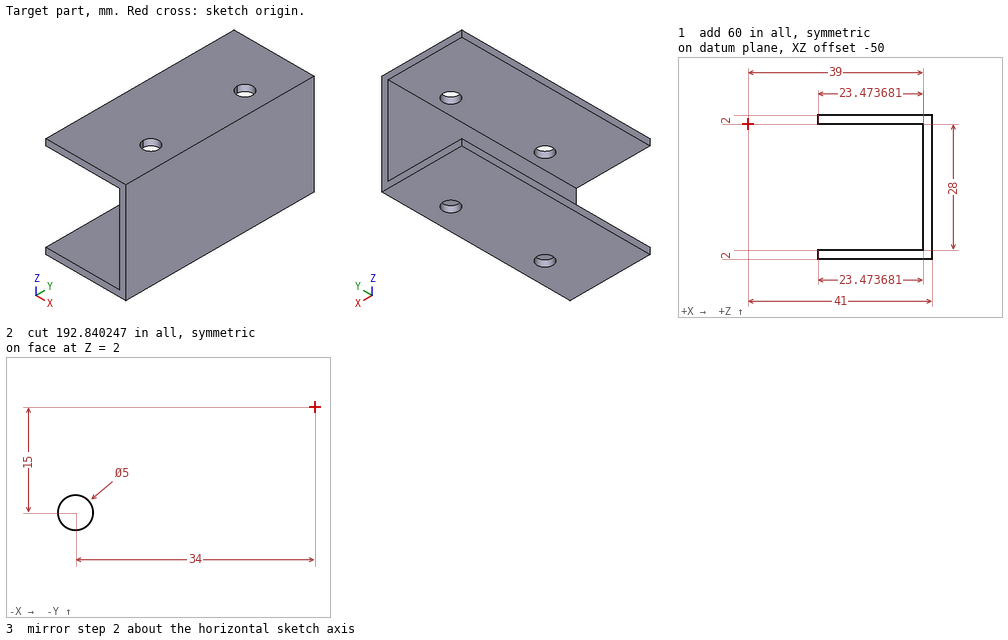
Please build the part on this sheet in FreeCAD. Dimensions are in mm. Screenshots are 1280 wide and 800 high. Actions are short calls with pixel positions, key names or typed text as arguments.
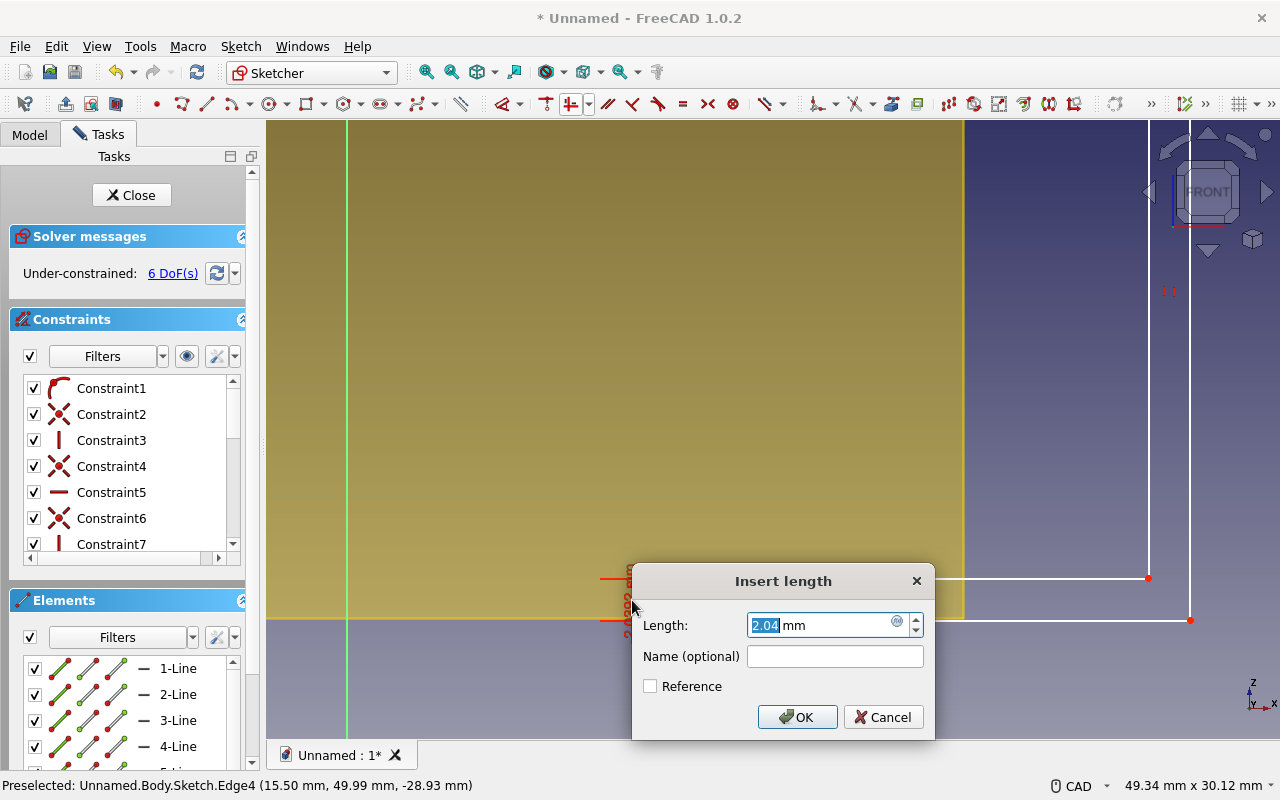
text(2)
key(Return)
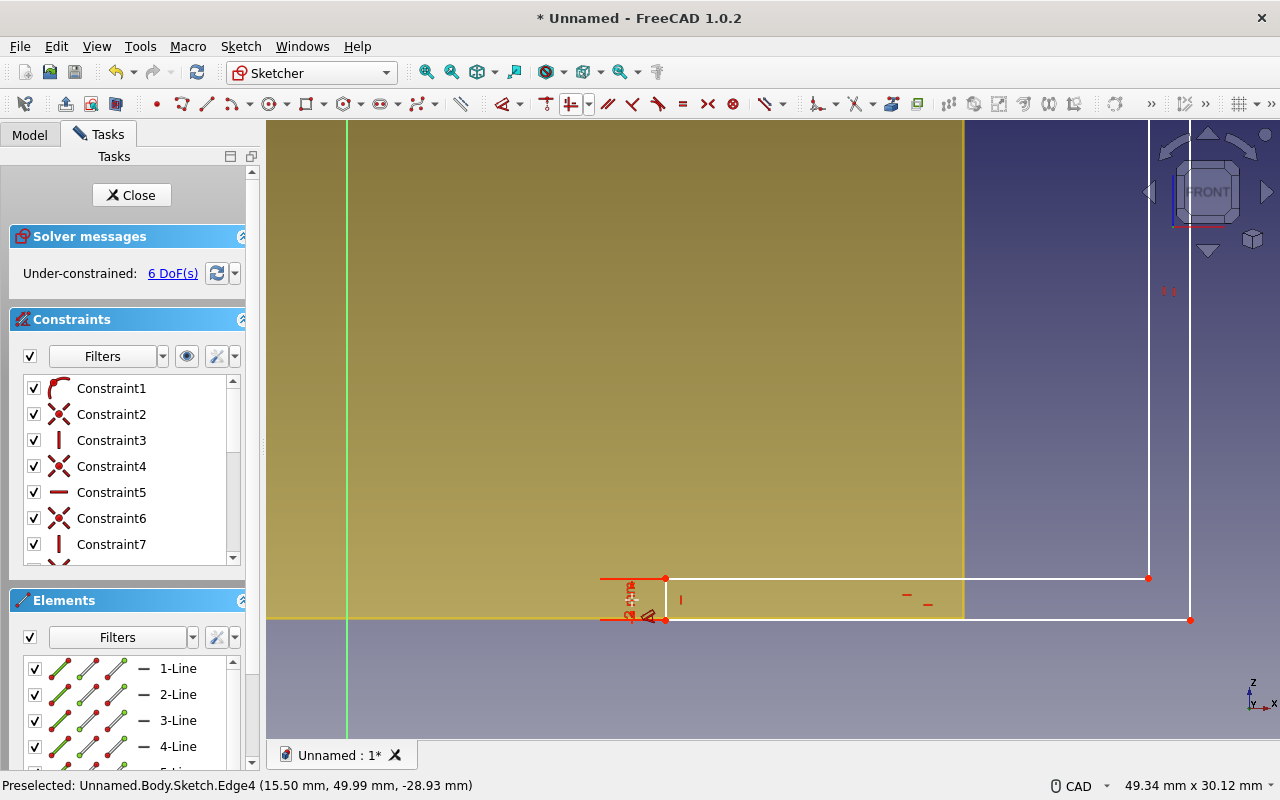
scroll(627, 599, down, 3)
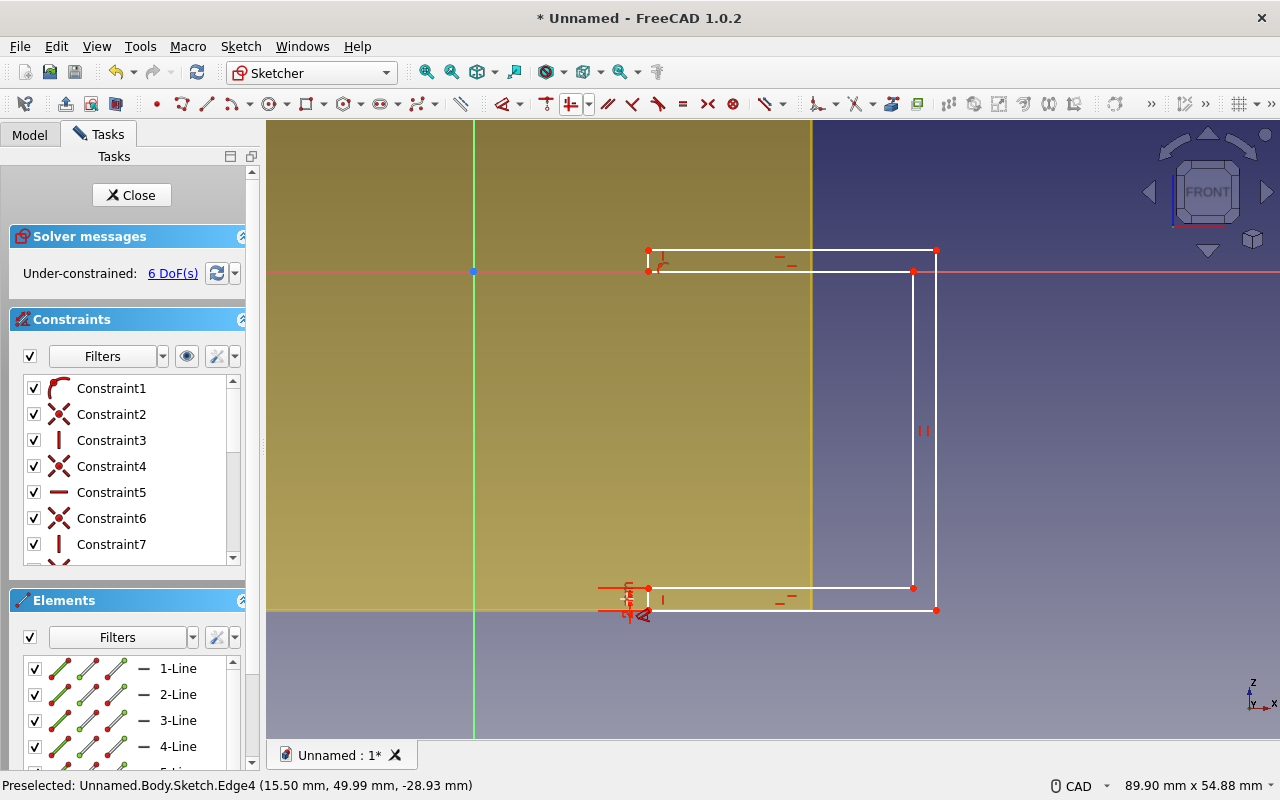
scroll(648, 257, up, 4)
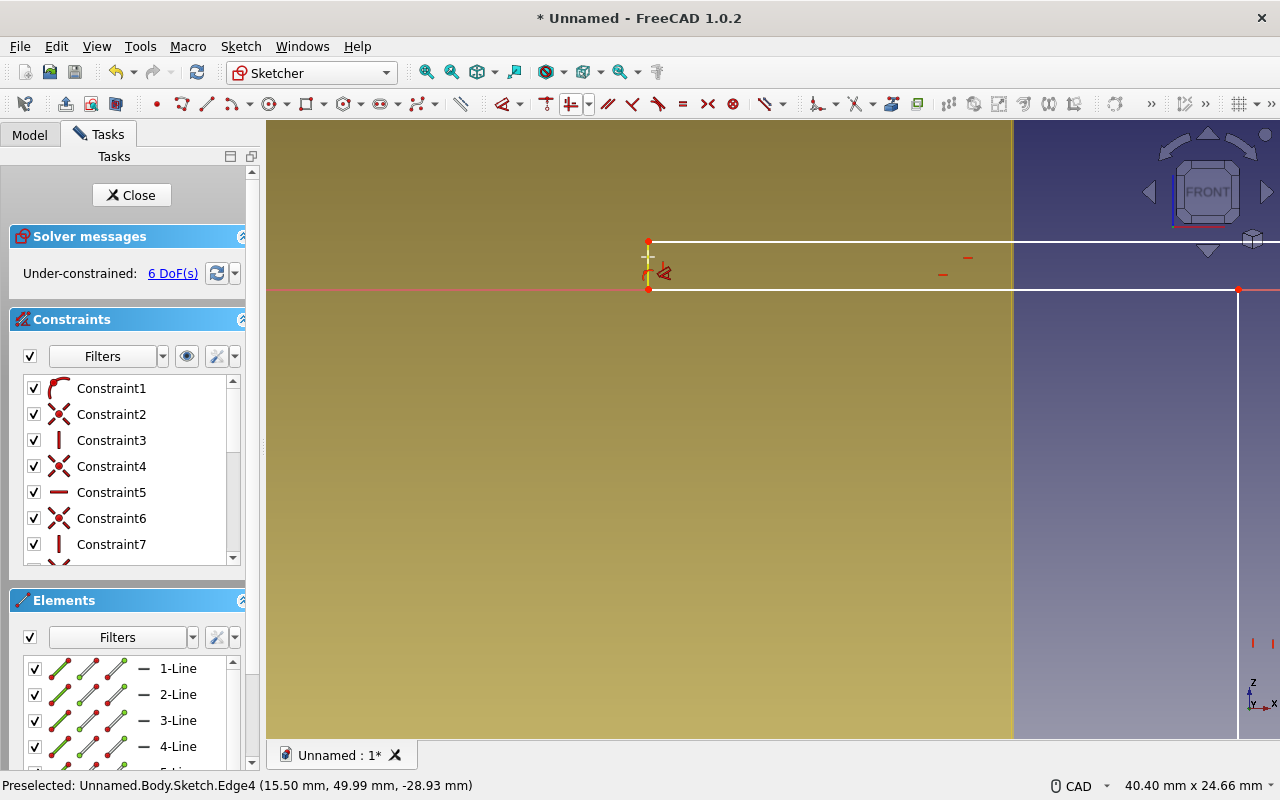
click(648, 256)
click(614, 266)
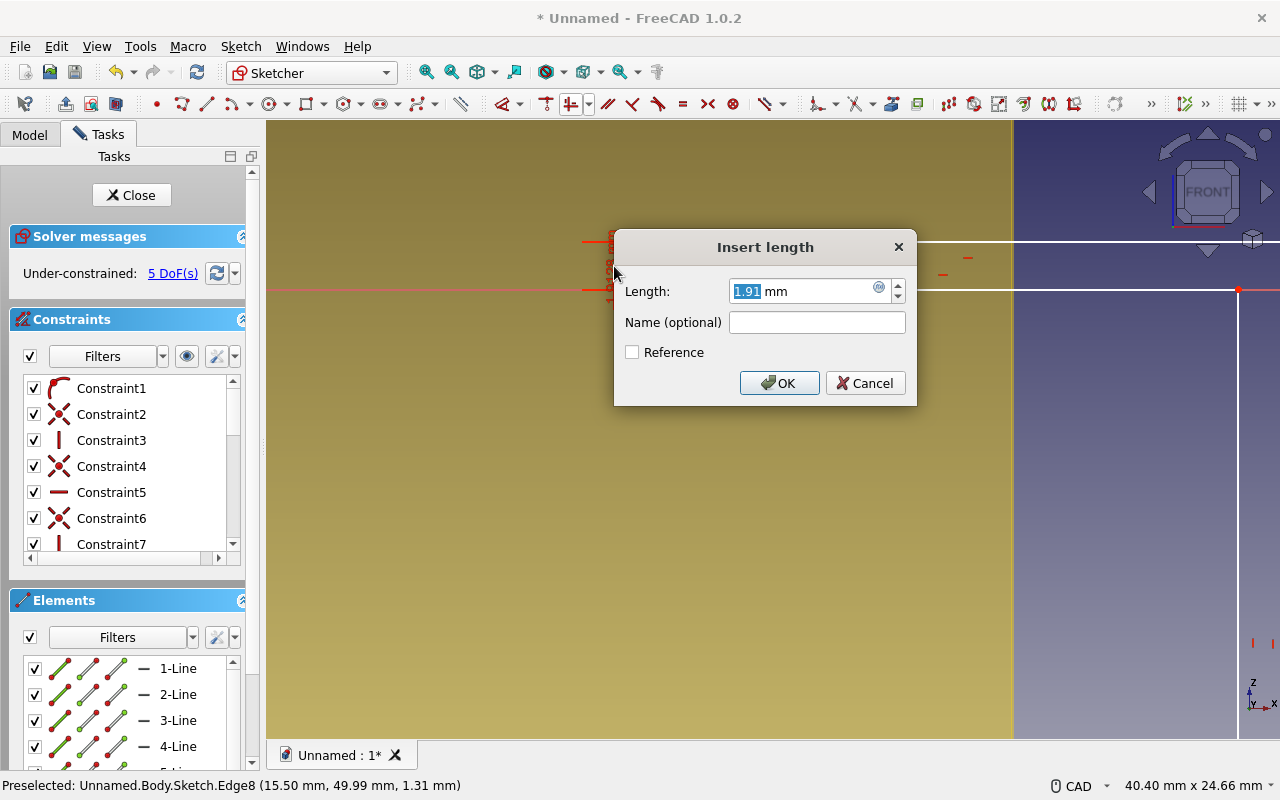
text(2)
key(Return)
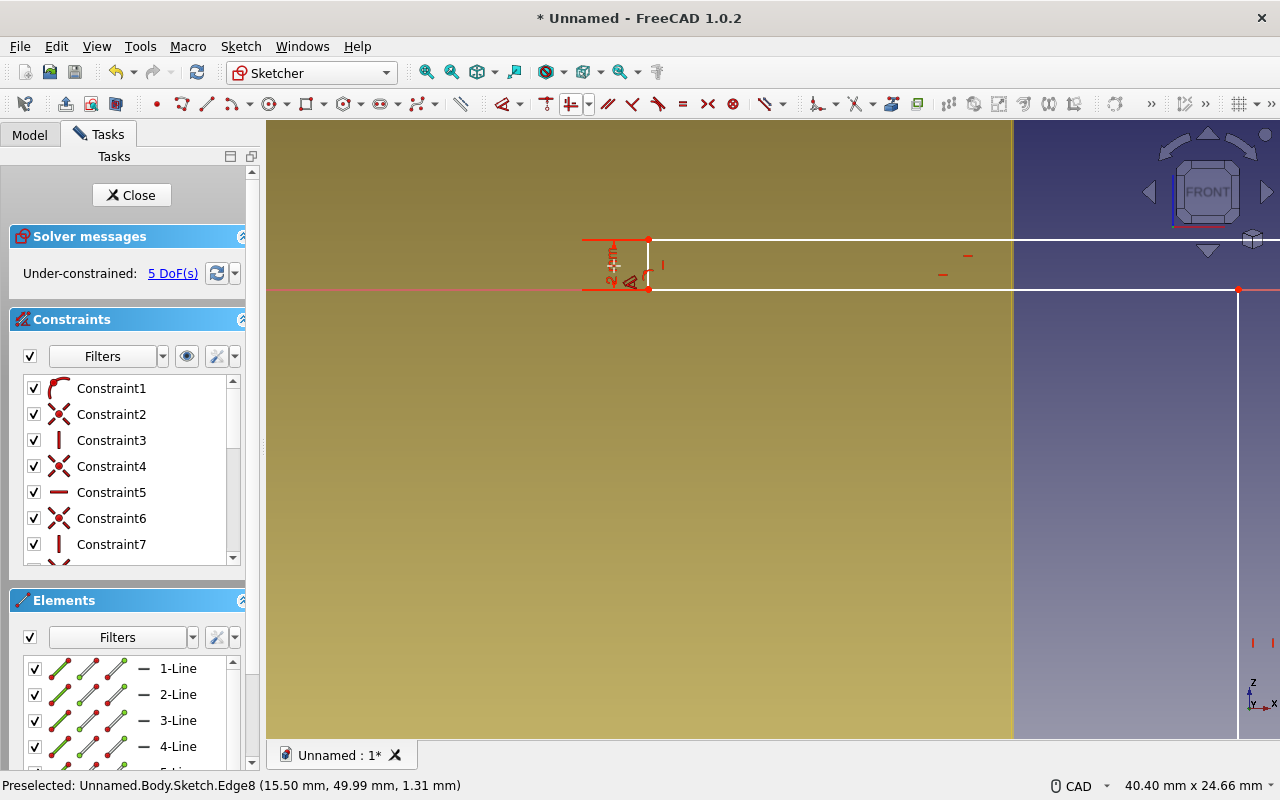
scroll(648, 257, down, 4)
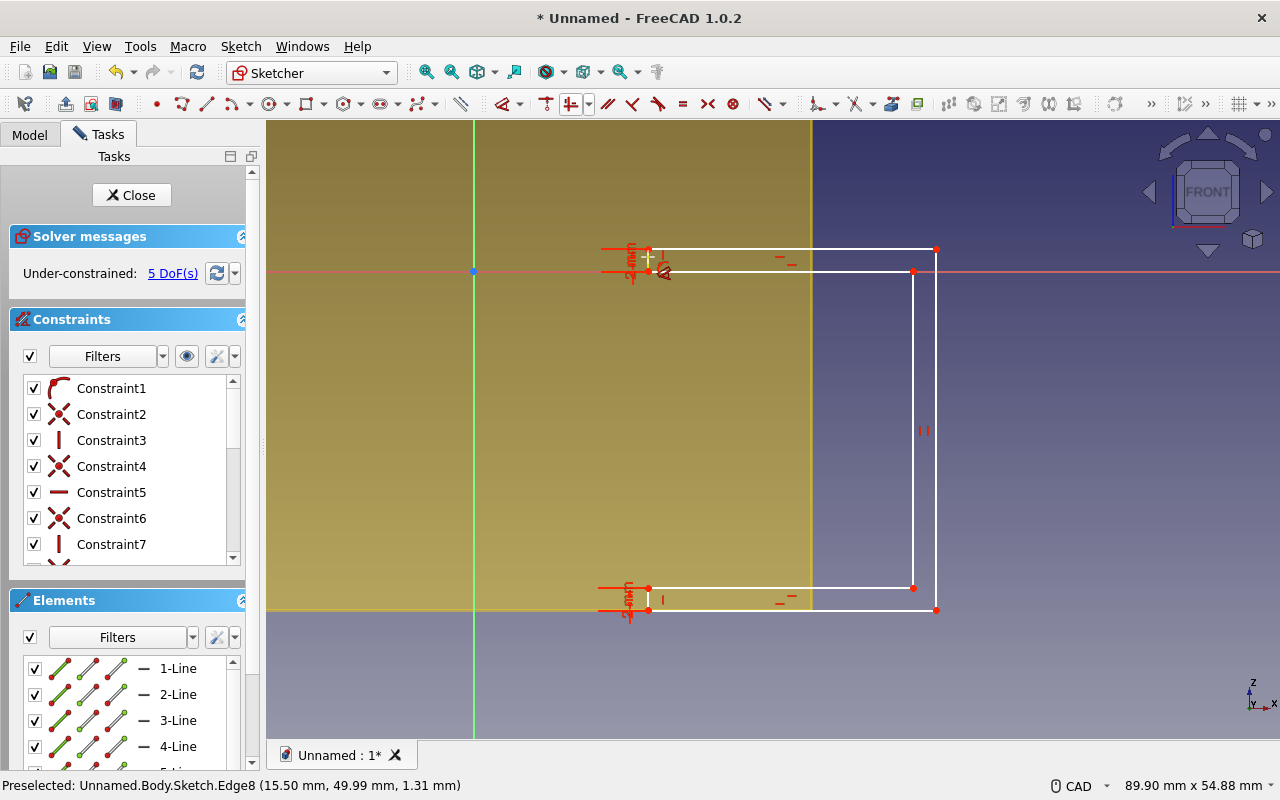
click(913, 367)
click(879, 430)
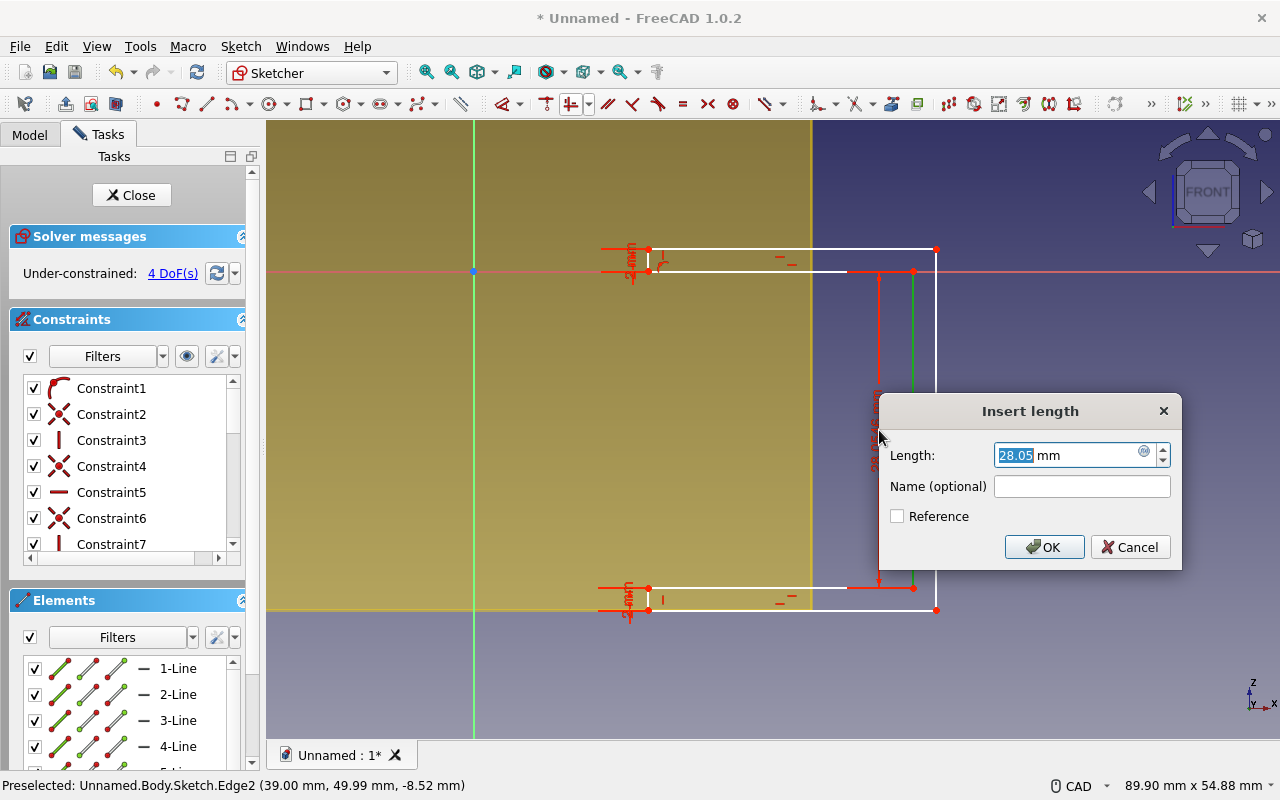
text(28)
key(Return)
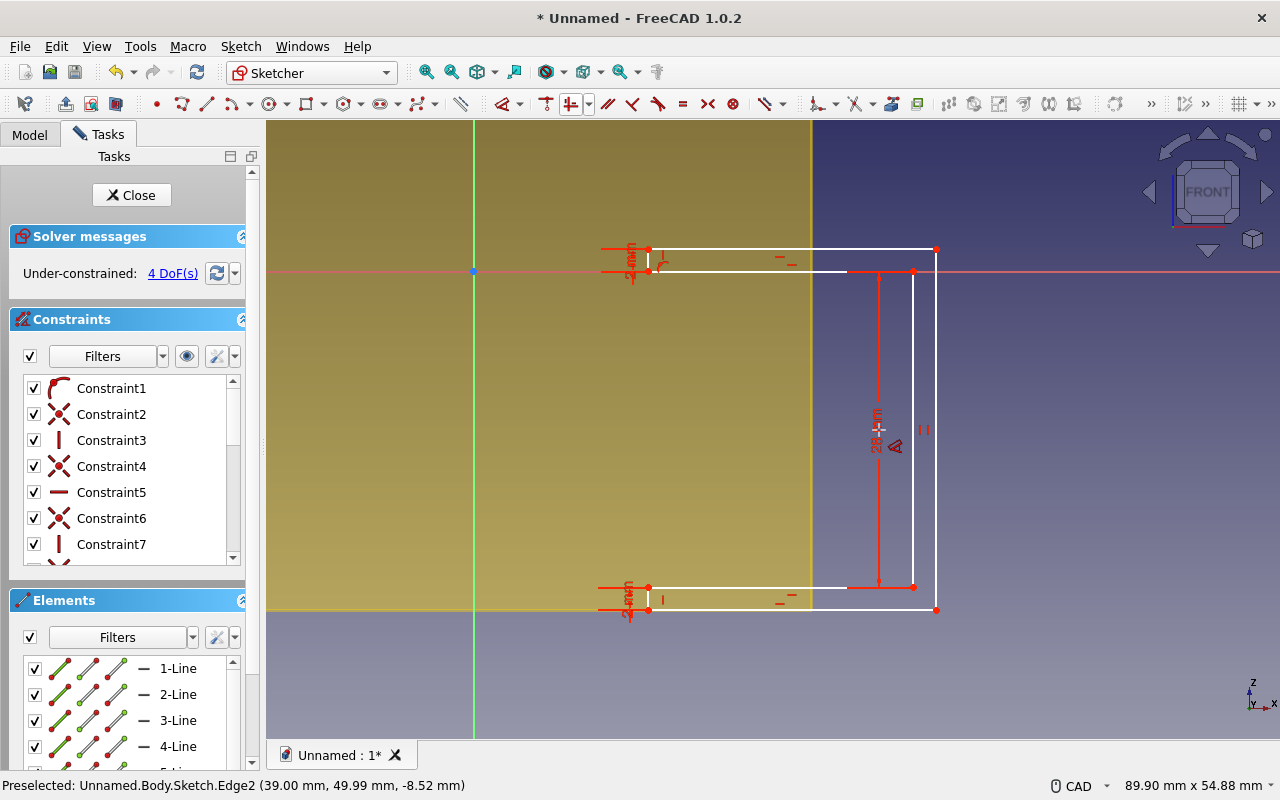
click(913, 272)
click(592, 238)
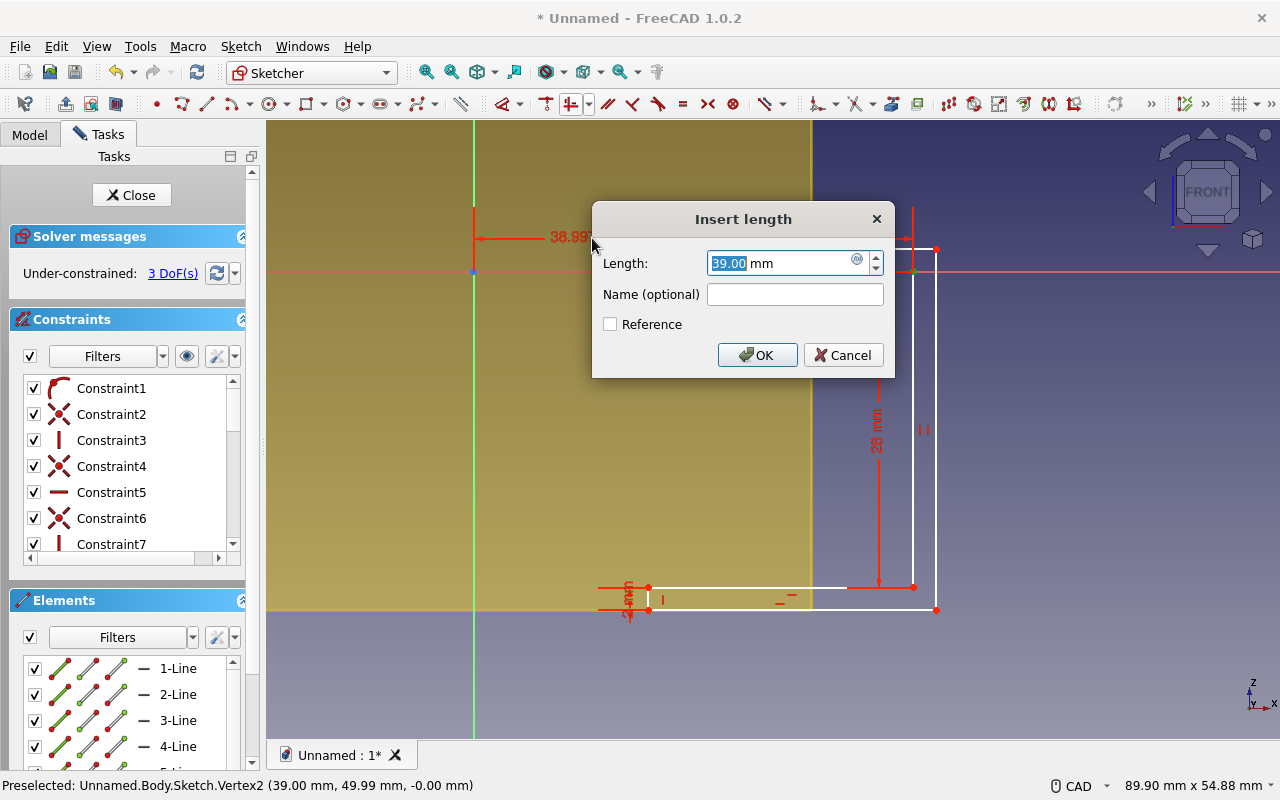
text(39)
key(Return)